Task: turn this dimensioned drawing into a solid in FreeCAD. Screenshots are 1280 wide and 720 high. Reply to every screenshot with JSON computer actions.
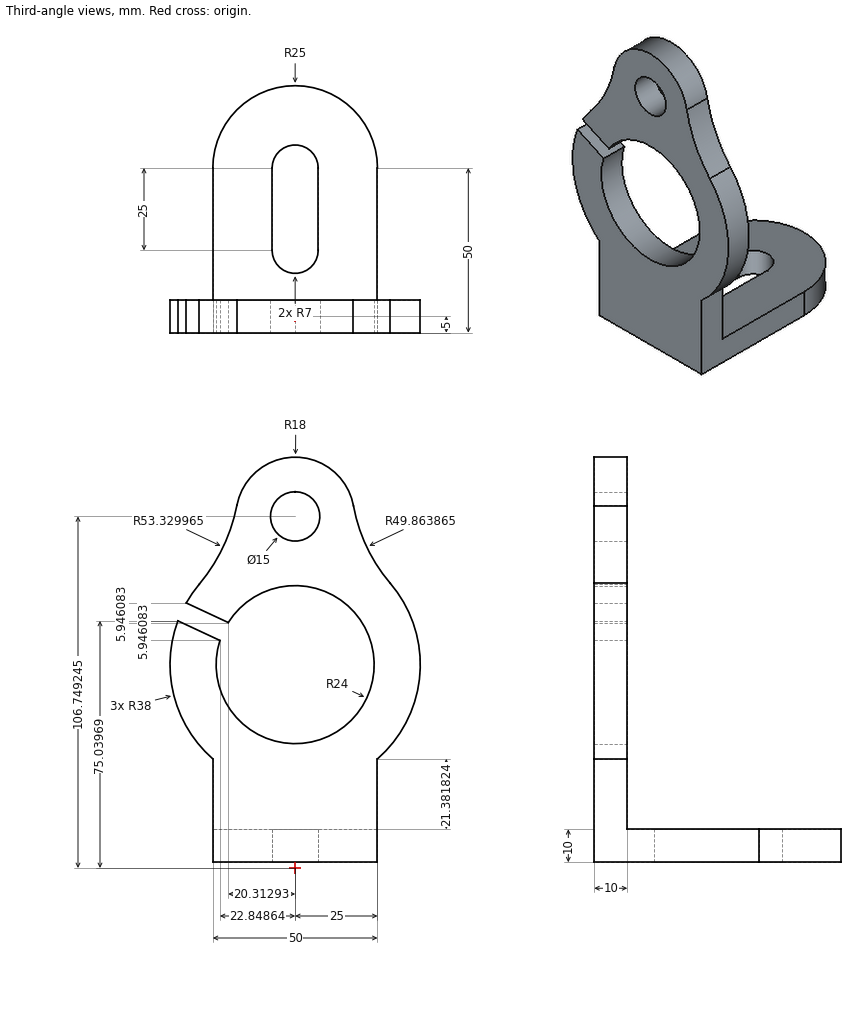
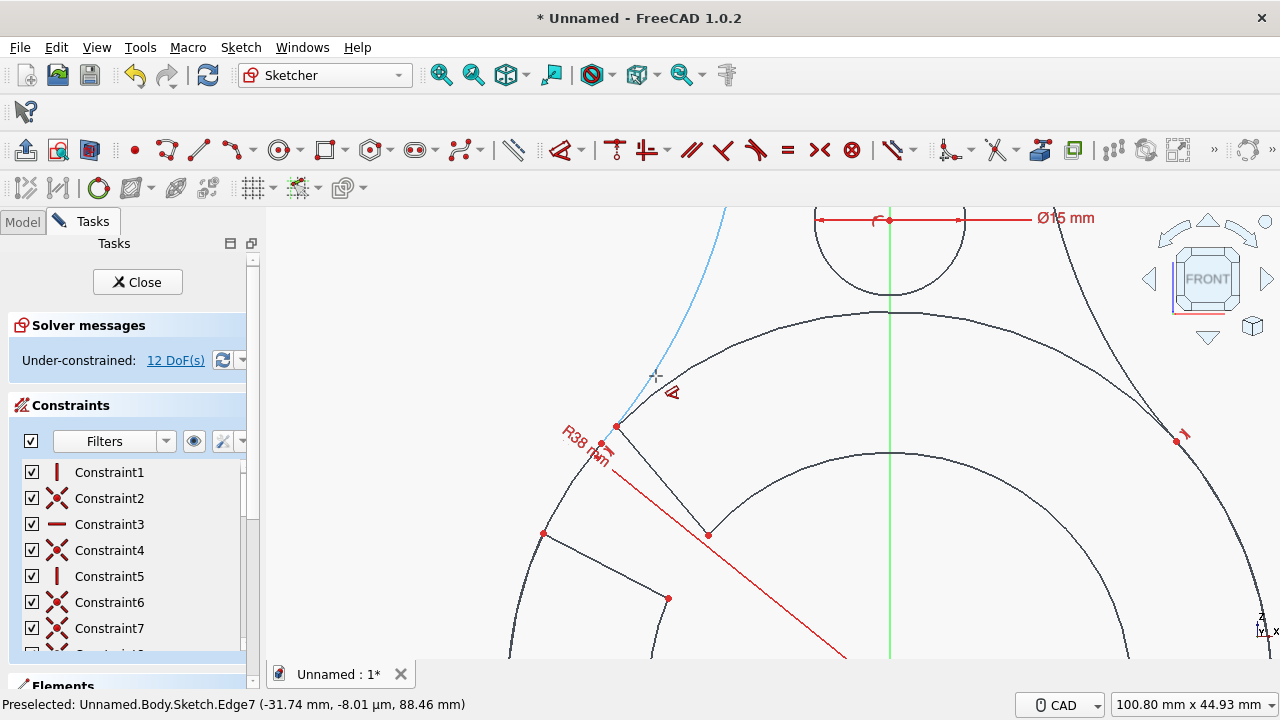
{"action": "left_click", "coordinate": [654, 373]}
{"action": "left_click", "coordinate": [681, 390]}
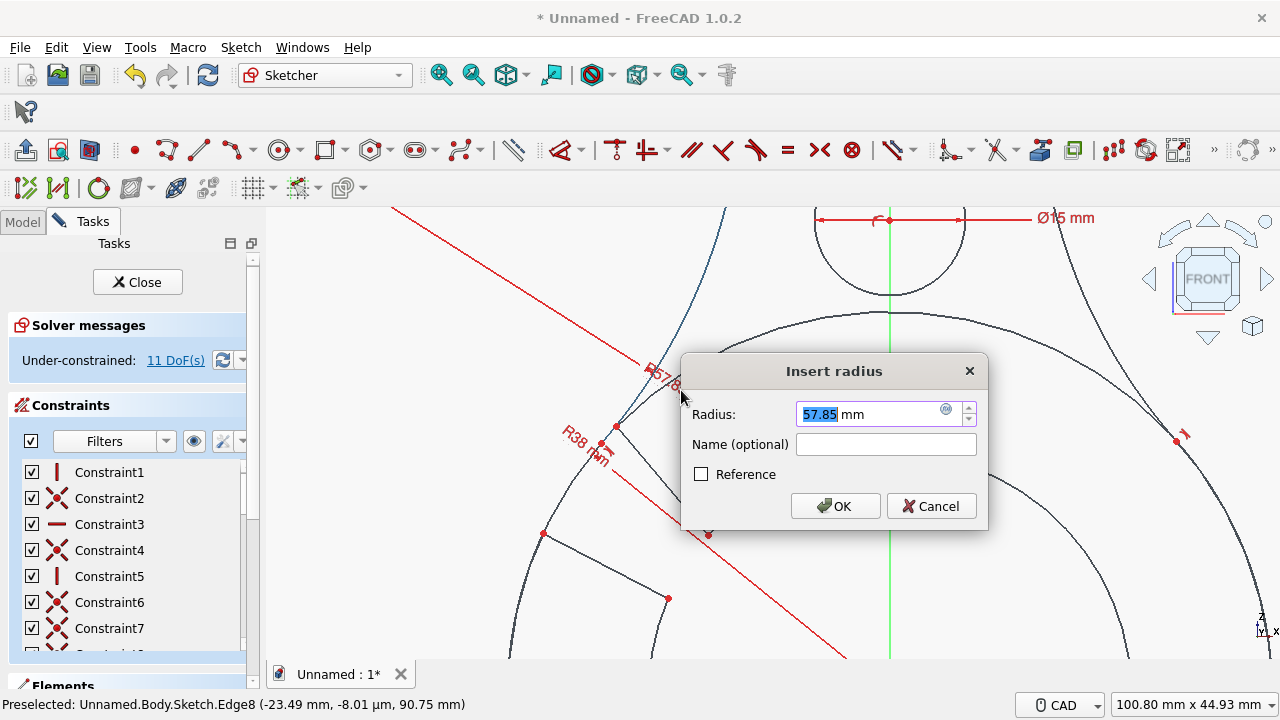
{"action": "type", "text": "53.329965"}
{"action": "key", "text": "Return"}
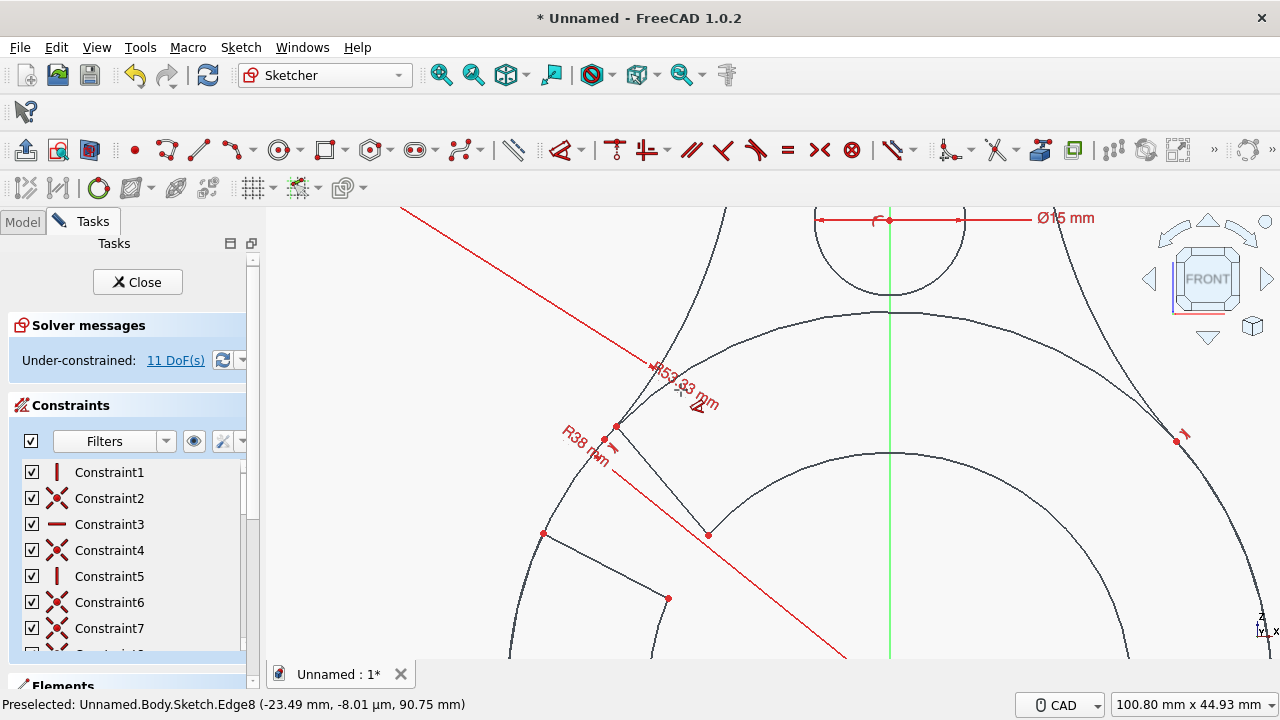
{"action": "scroll", "coordinate": [656, 376], "scroll_direction": "down", "scroll_amount": 8}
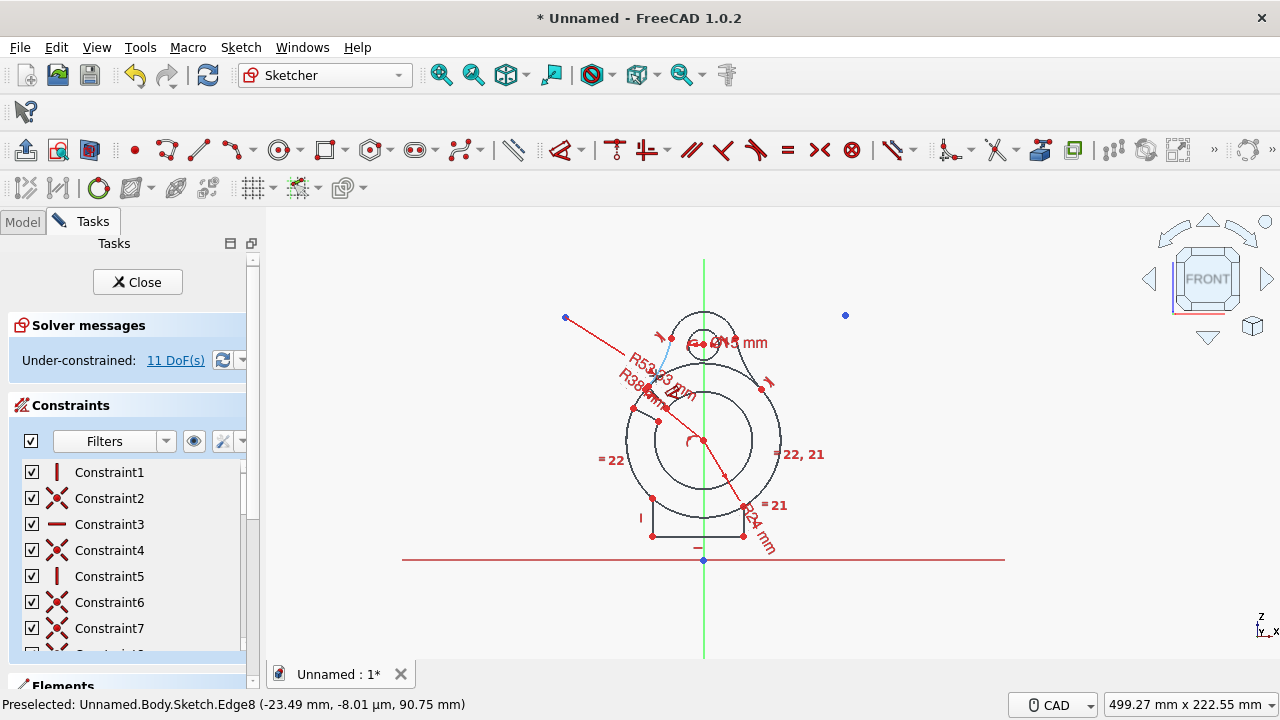
{"action": "left_click", "coordinate": [721, 317]}
{"action": "left_click", "coordinate": [738, 290]}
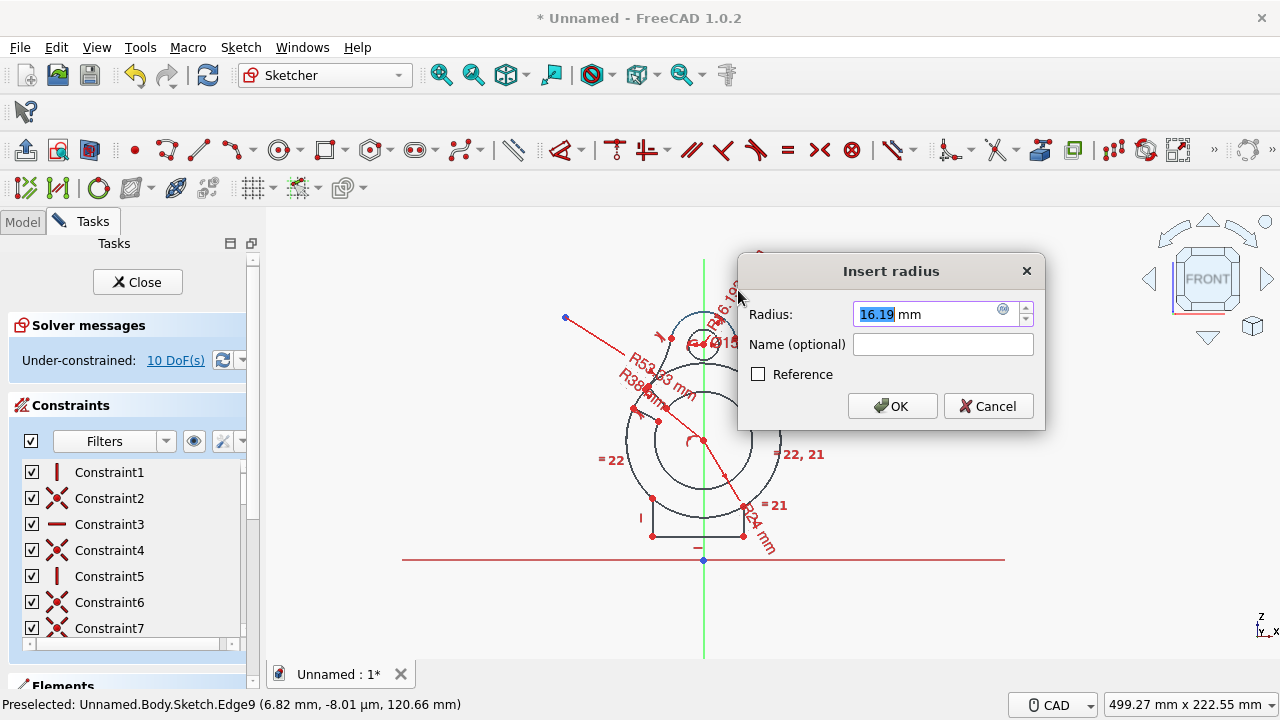
{"action": "type", "text": "18"}
{"action": "key", "text": "Return"}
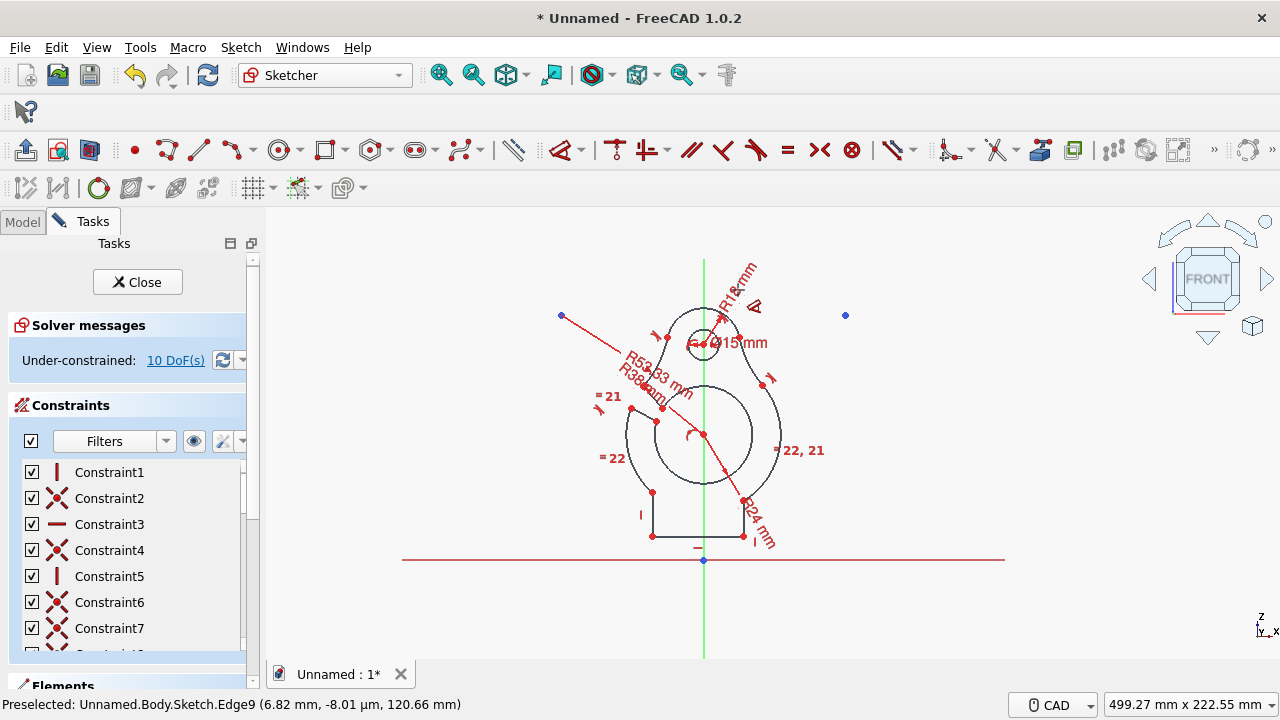
{"action": "left_click", "coordinate": [744, 353]}
{"action": "left_click", "coordinate": [816, 452]}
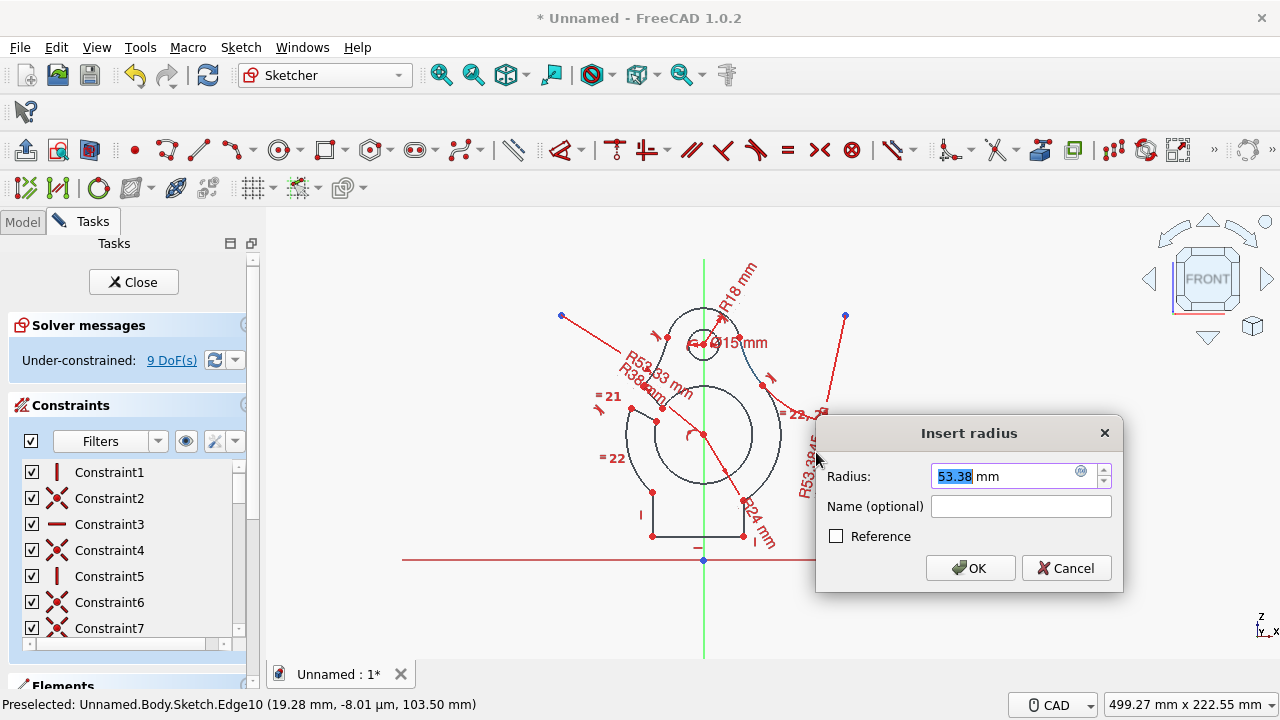
{"action": "type", "text": "49.863865"}
{"action": "key", "text": "Return"}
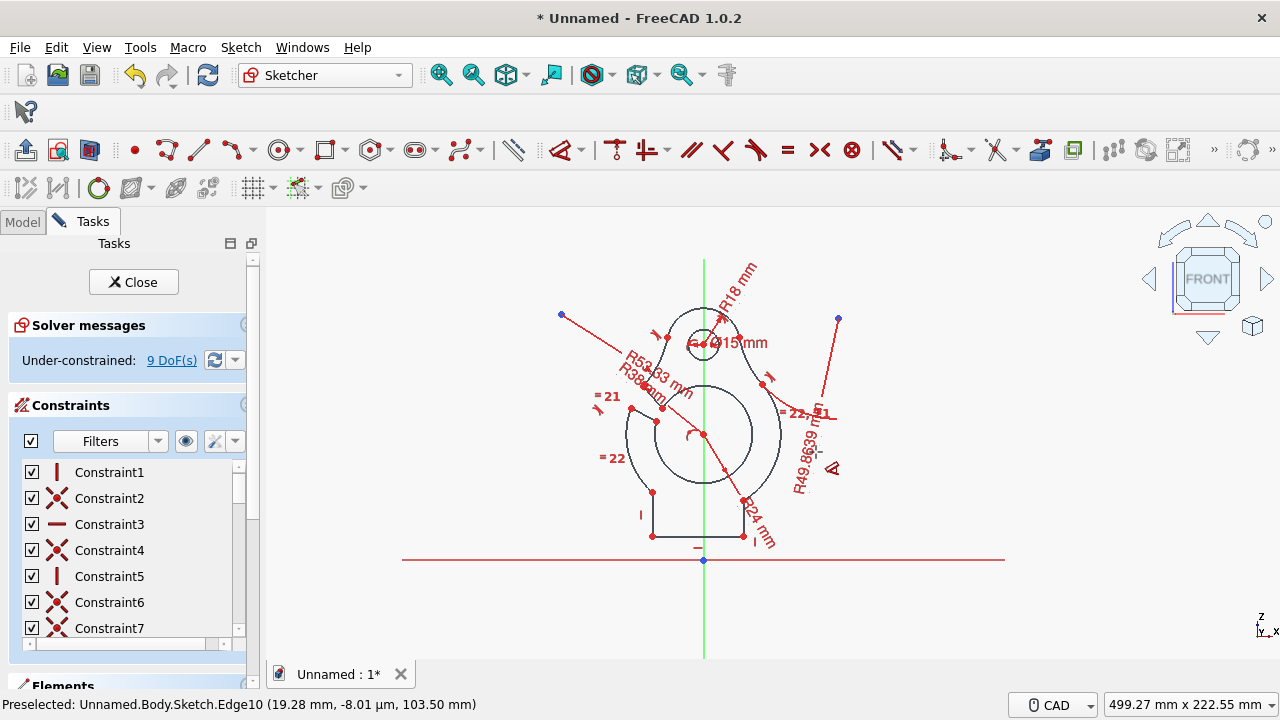
{"action": "left_click", "coordinate": [717, 537]}
{"action": "left_click", "coordinate": [677, 503]}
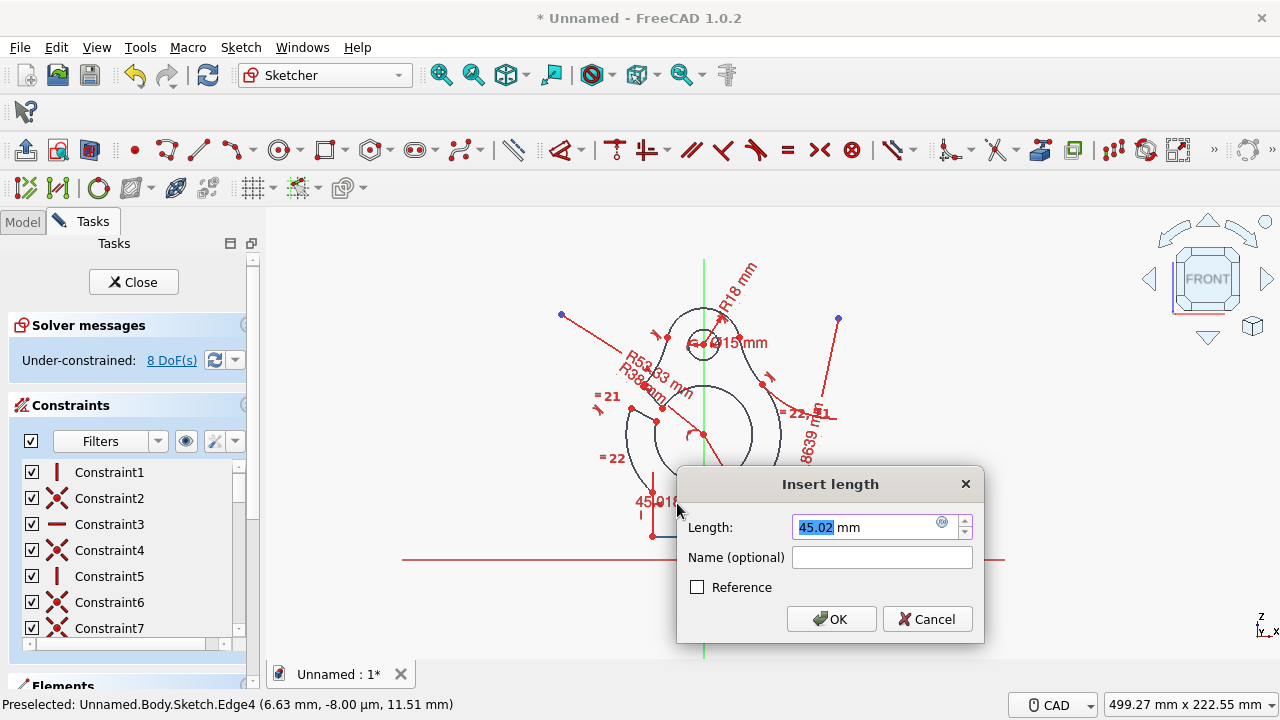
{"action": "type", "text": "50"}
{"action": "key", "text": "Return"}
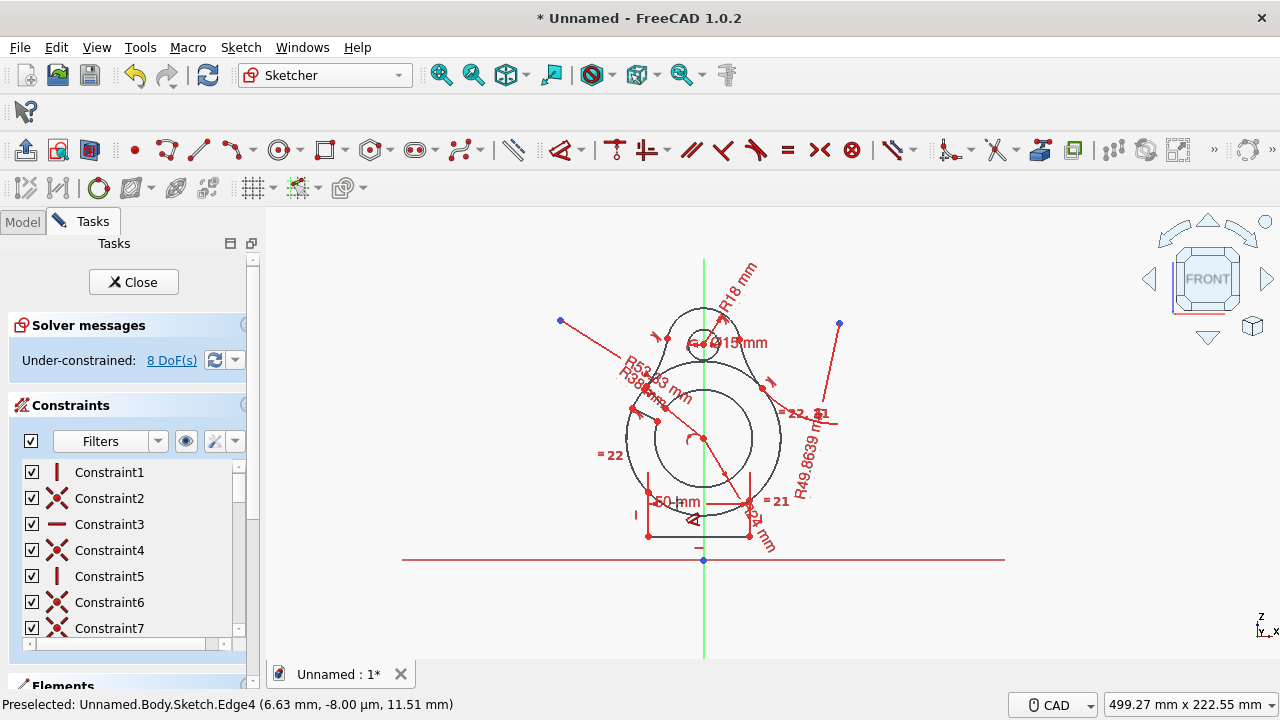
{"action": "left_click", "coordinate": [750, 500]}
{"action": "left_click", "coordinate": [727, 594]}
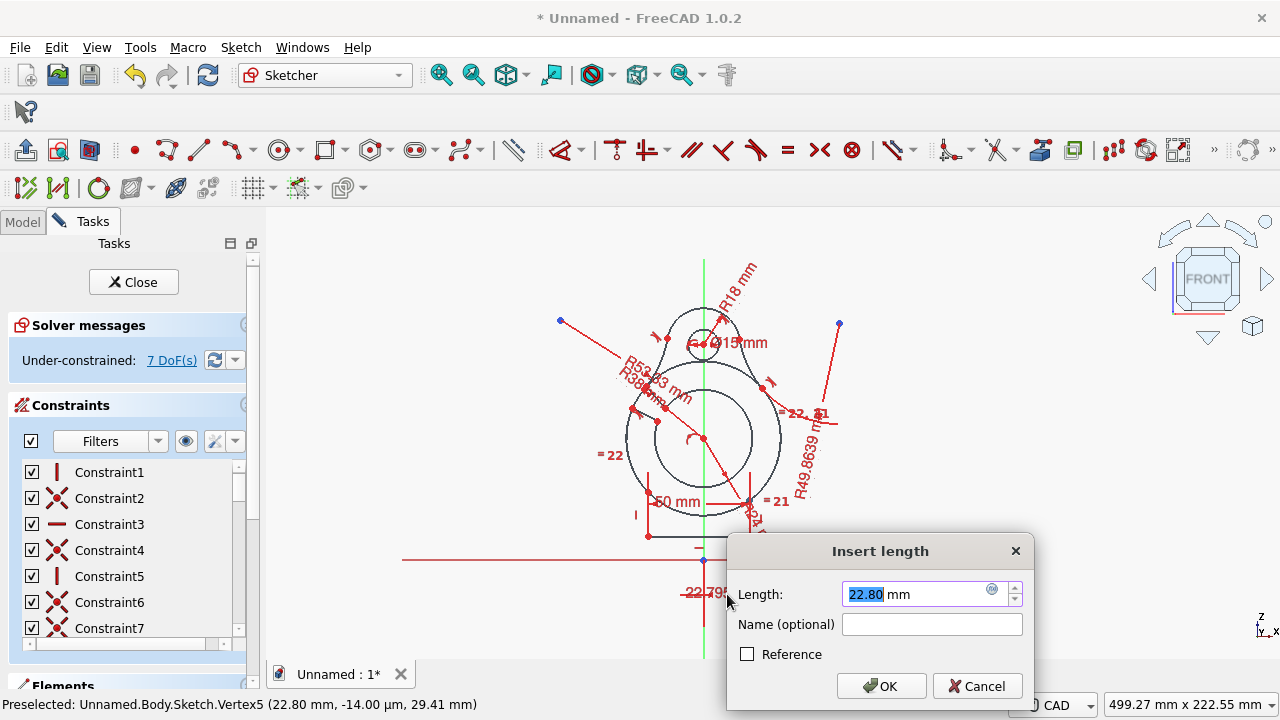
{"action": "type", "text": "25"}
{"action": "key", "text": "Return"}